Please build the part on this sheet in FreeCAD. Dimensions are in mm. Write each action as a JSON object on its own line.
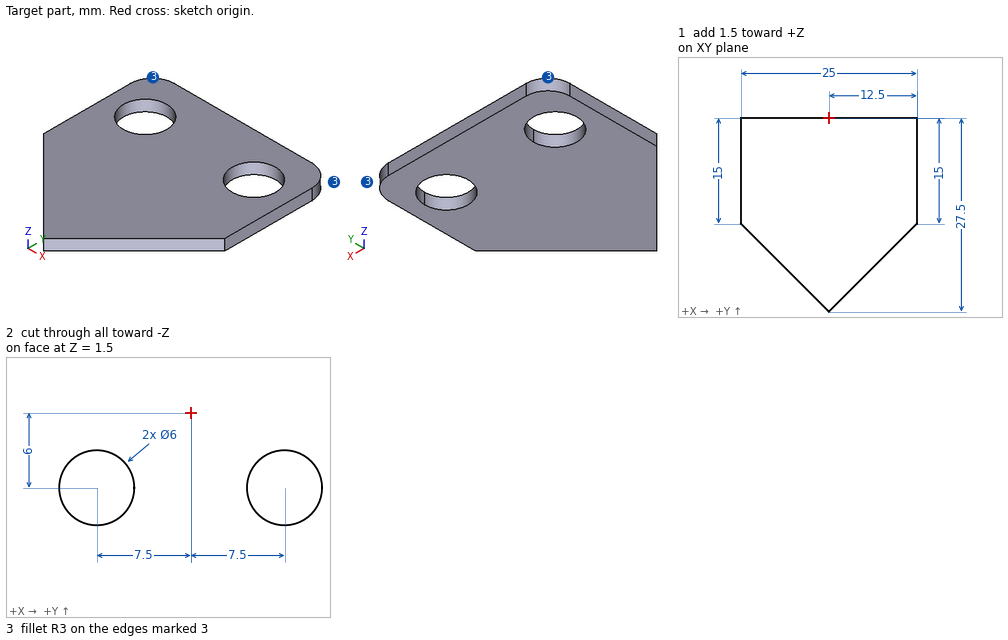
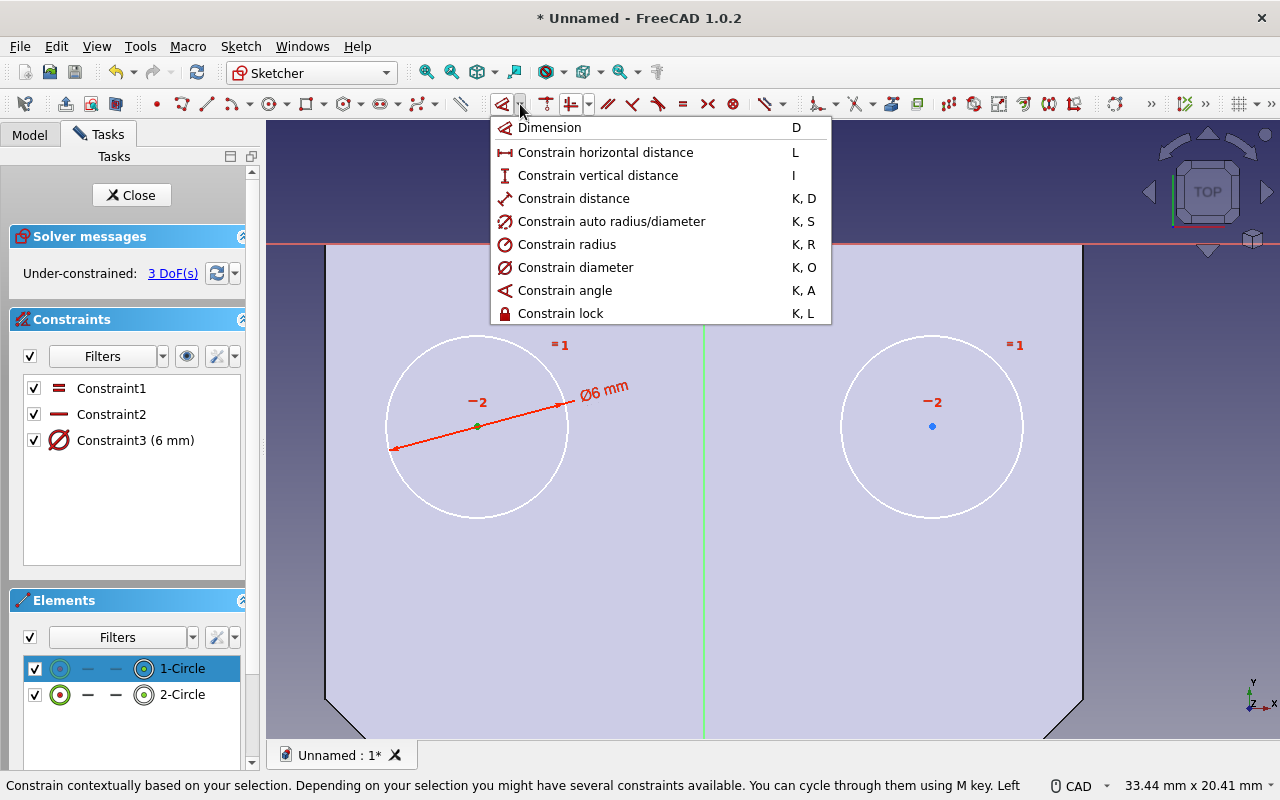
{"action": "left_click", "coordinate": [661, 176]}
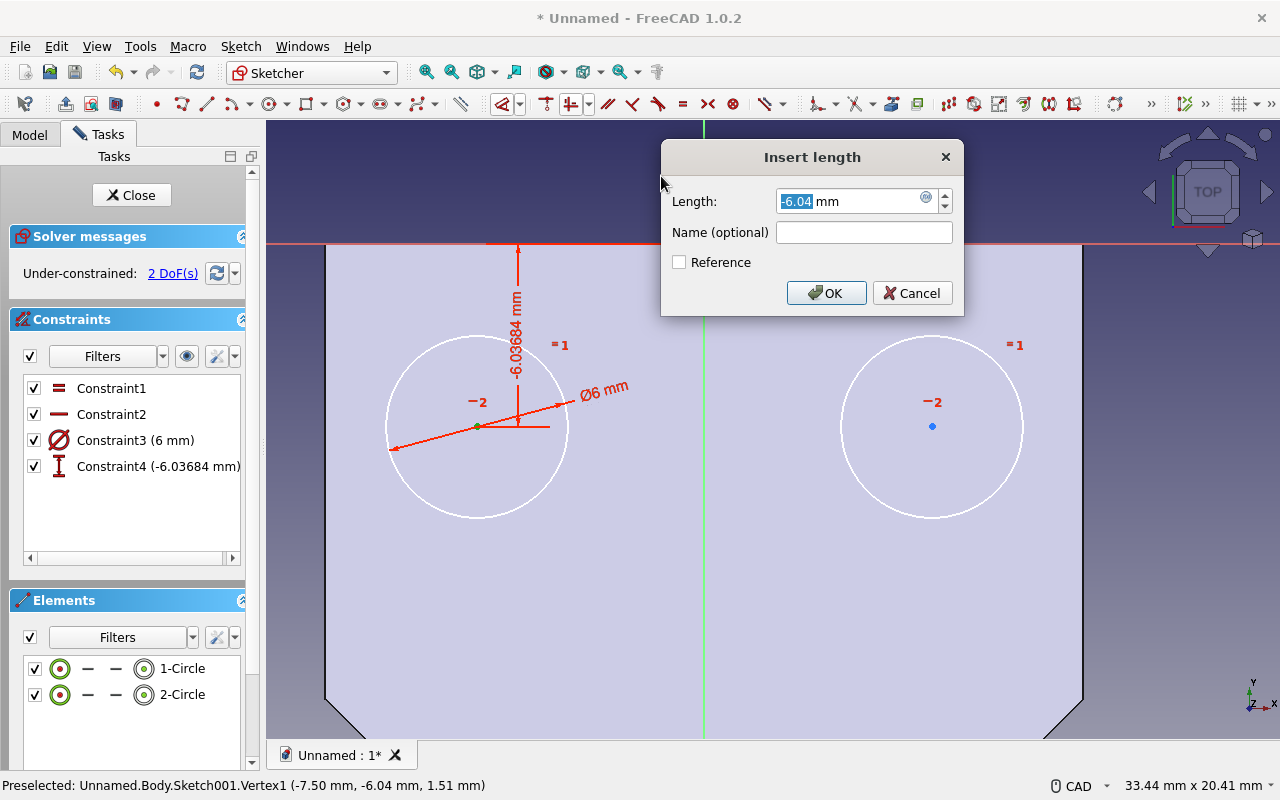
{"action": "type", "text": "-6"}
{"action": "key", "text": "Return"}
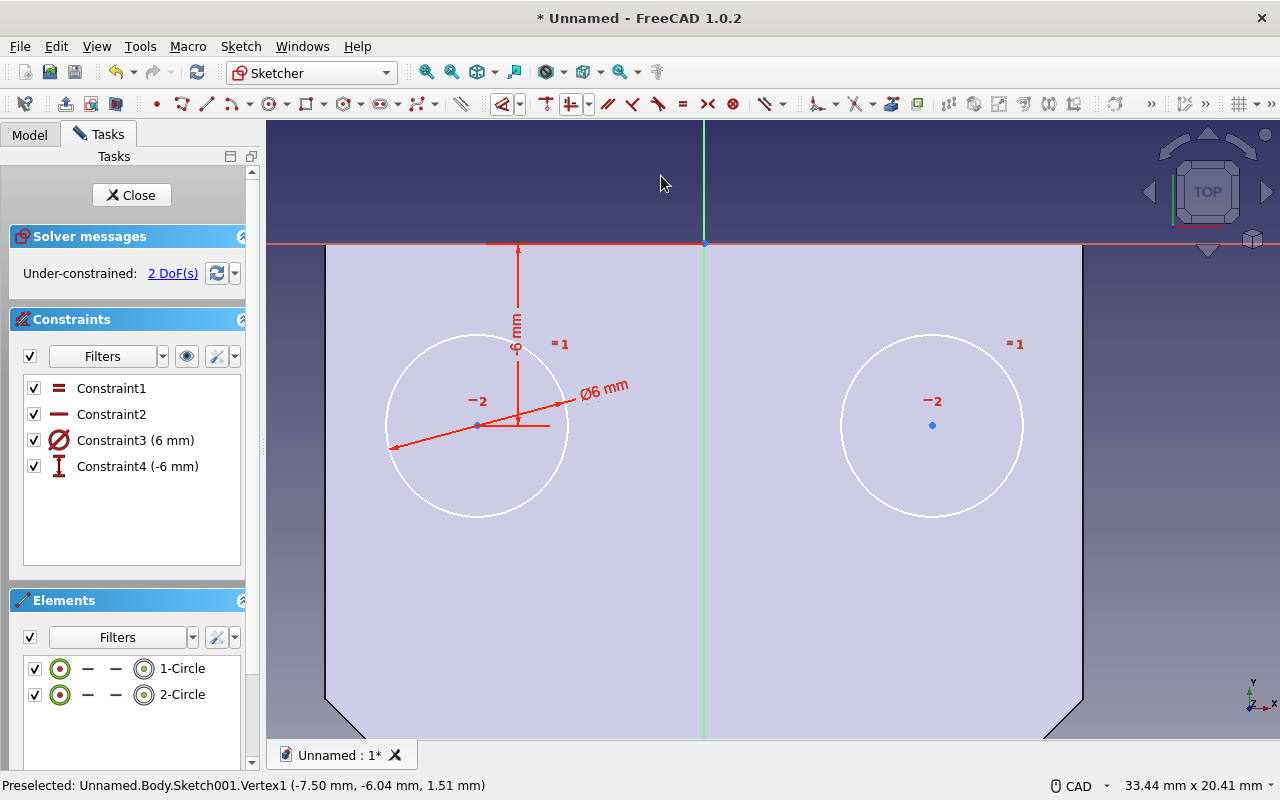
{"action": "left_click", "coordinate": [477, 426]}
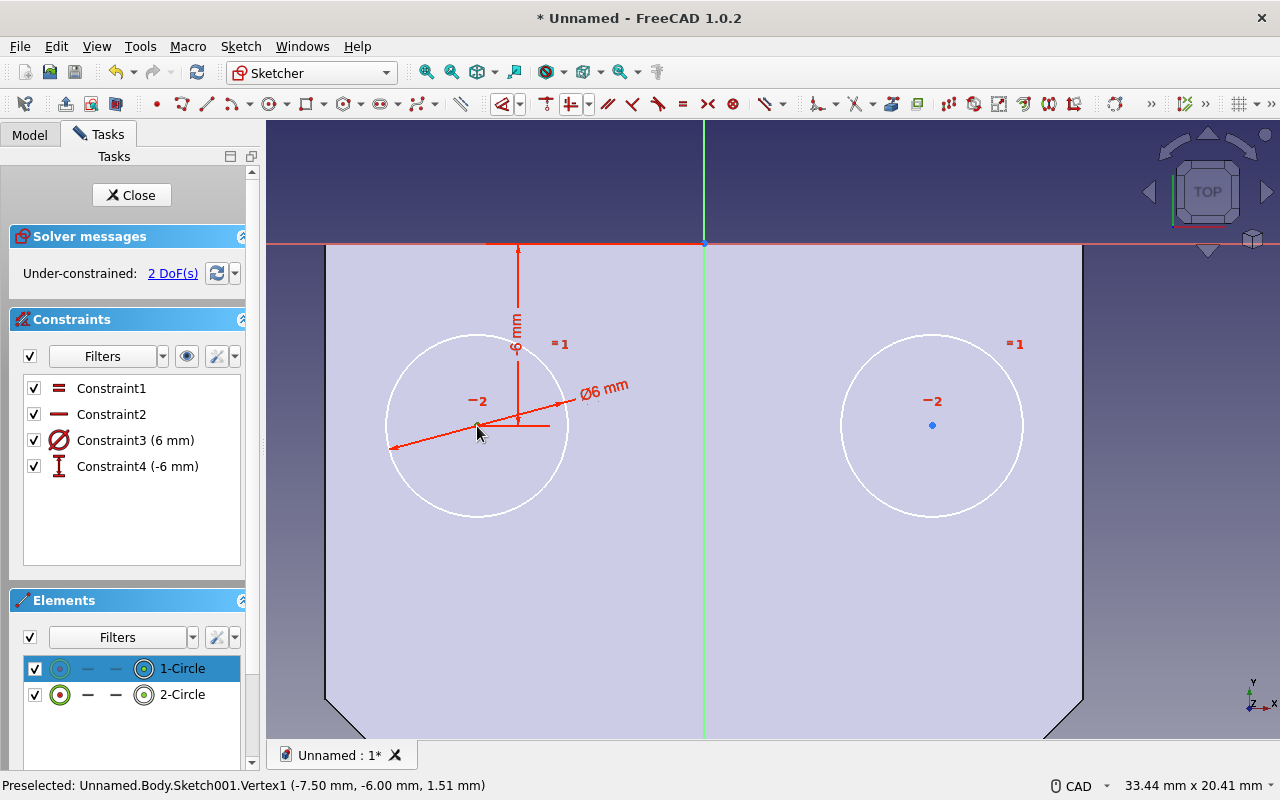
{"action": "left_click", "coordinate": [520, 104]}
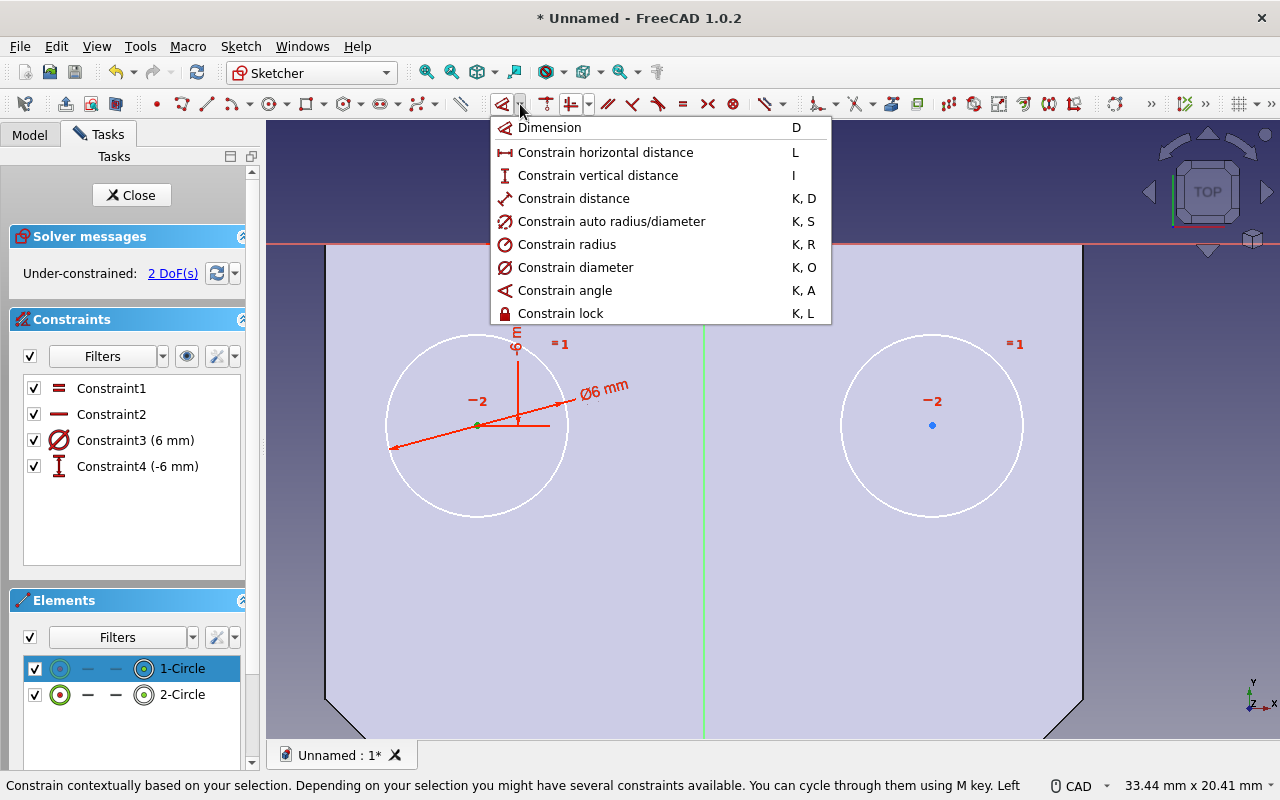
{"action": "left_click", "coordinate": [661, 152]}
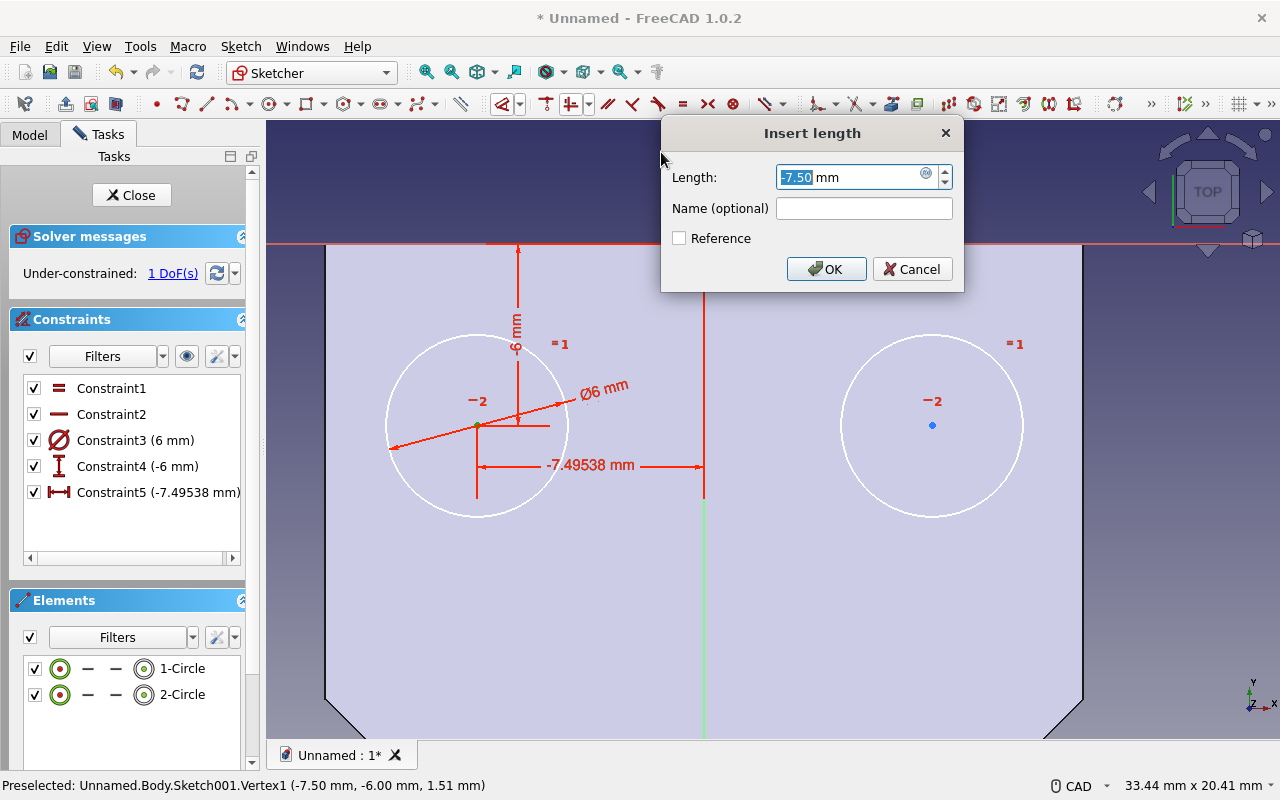
{"action": "type", "text": "-7.5"}
{"action": "key", "text": "Return"}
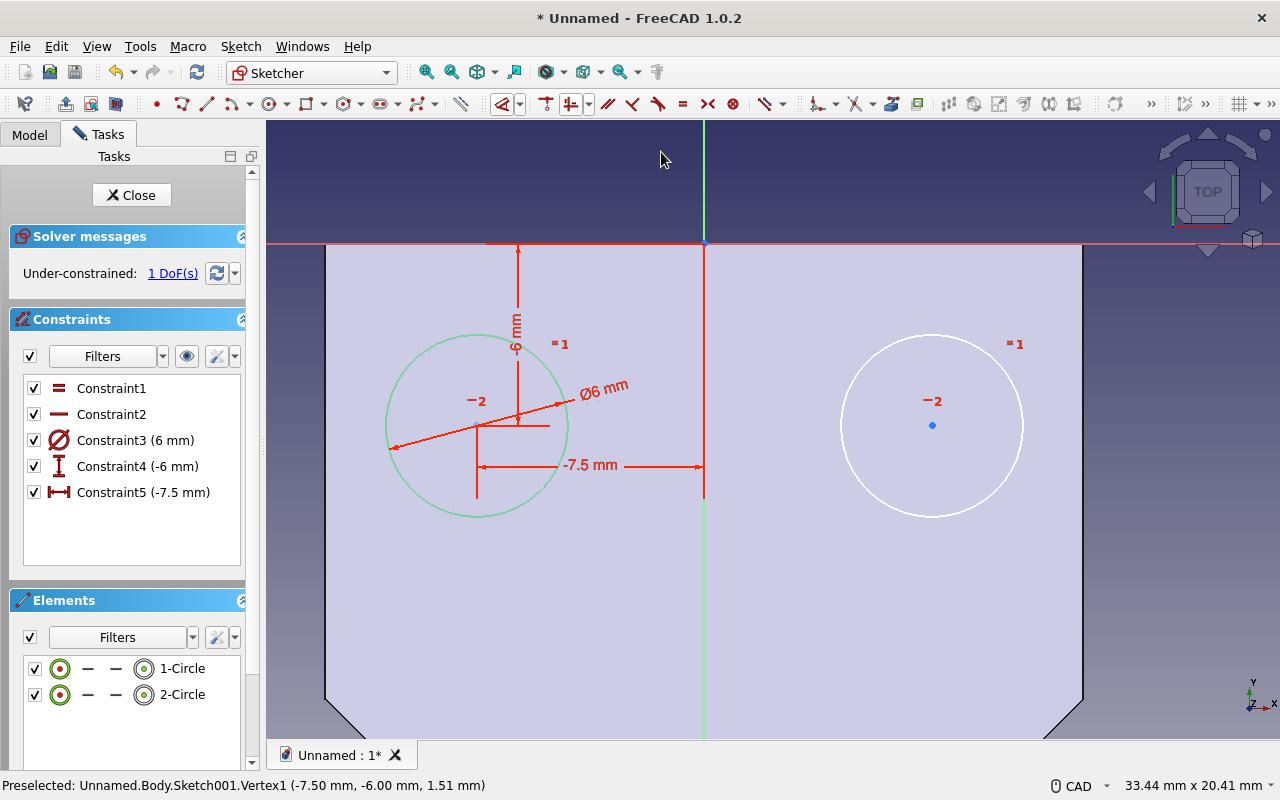
{"action": "left_click", "coordinate": [932, 426]}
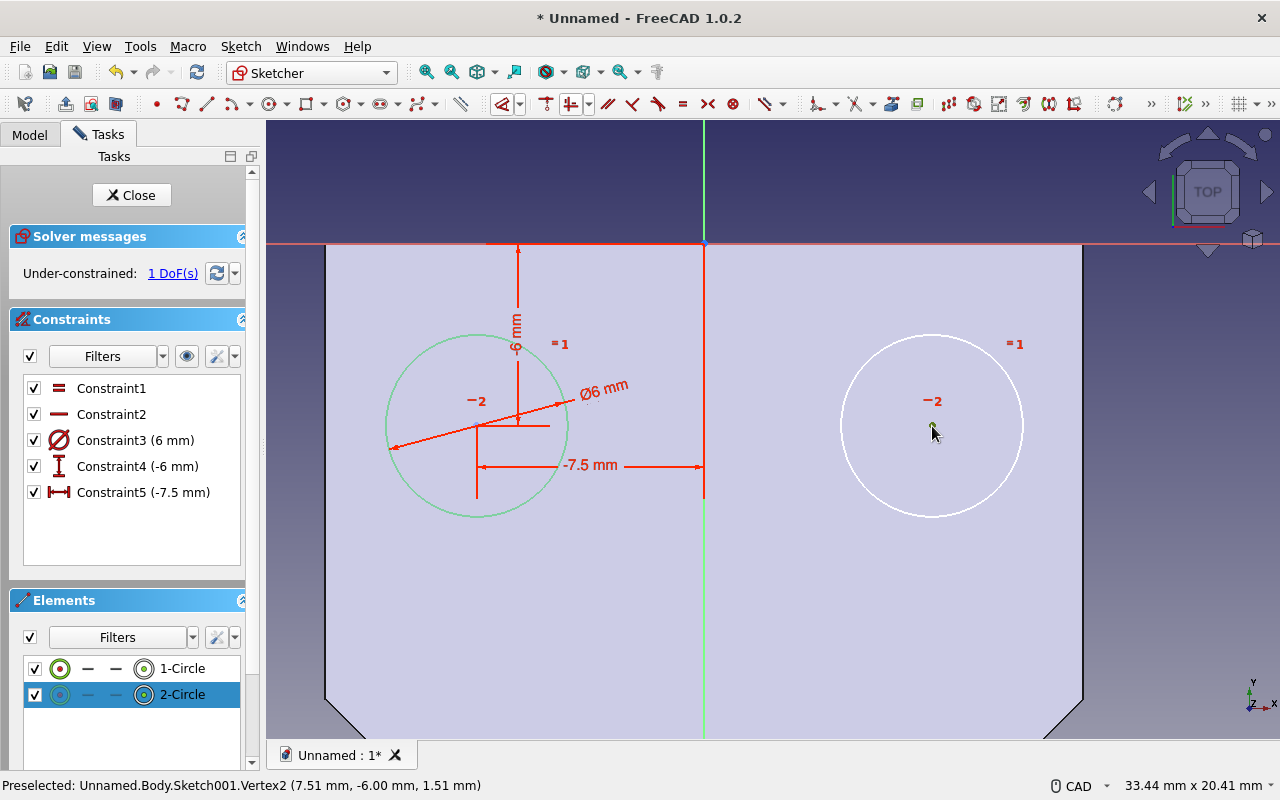
{"action": "left_click", "coordinate": [520, 104]}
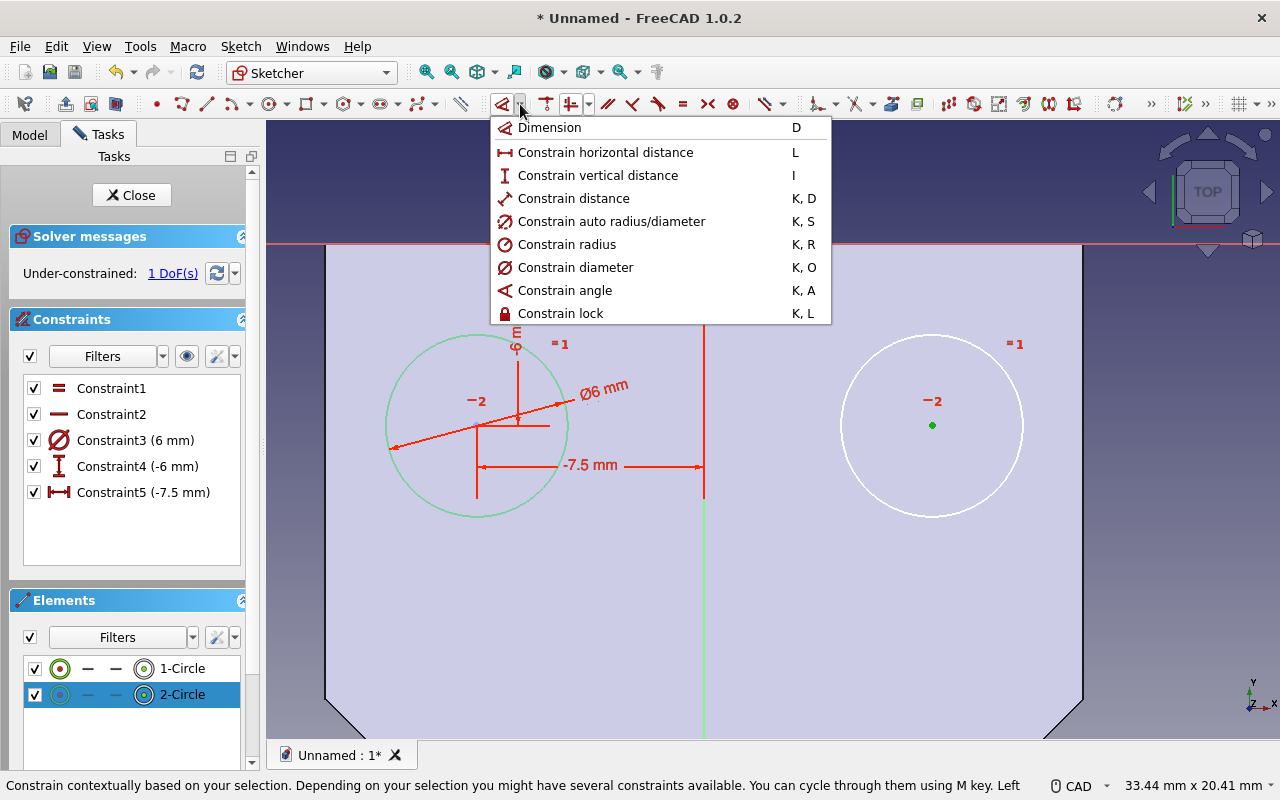
{"action": "left_click", "coordinate": [661, 152]}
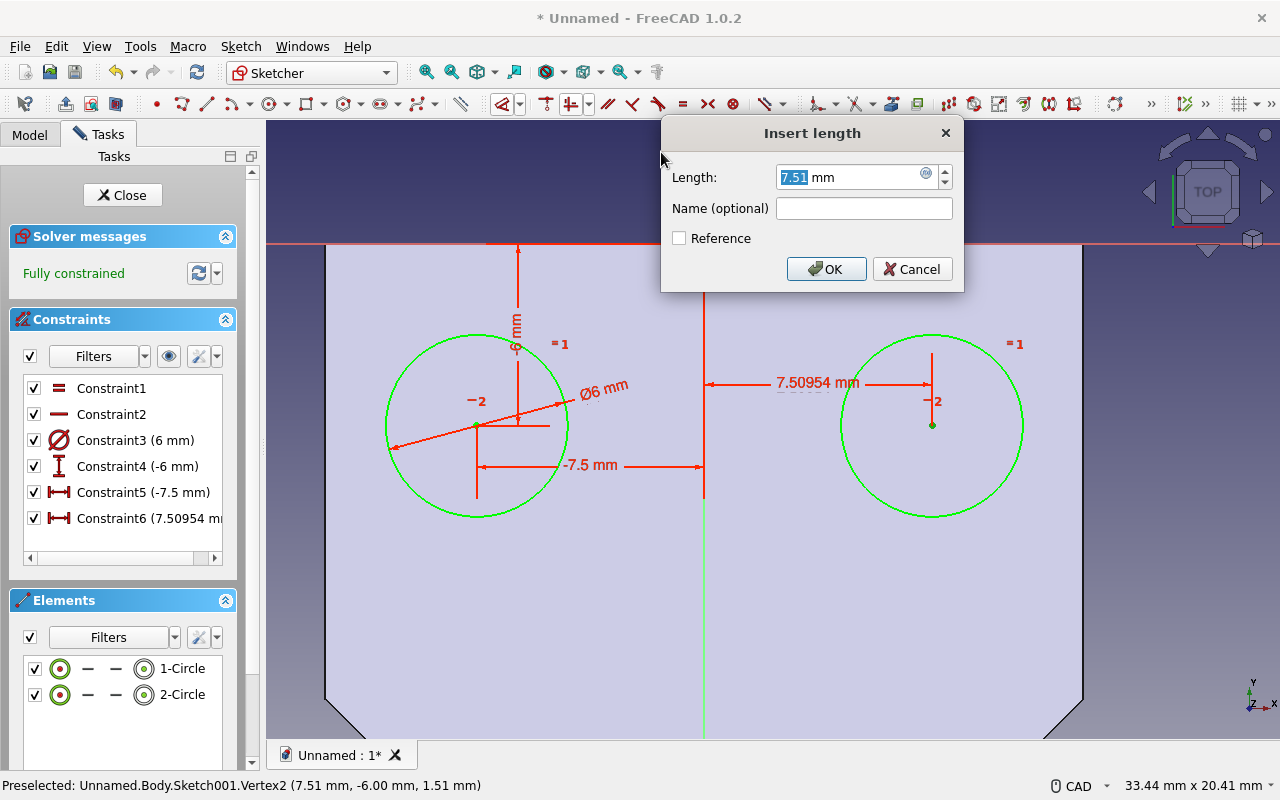
{"action": "type", "text": "7.5"}
{"action": "key", "text": "Return"}